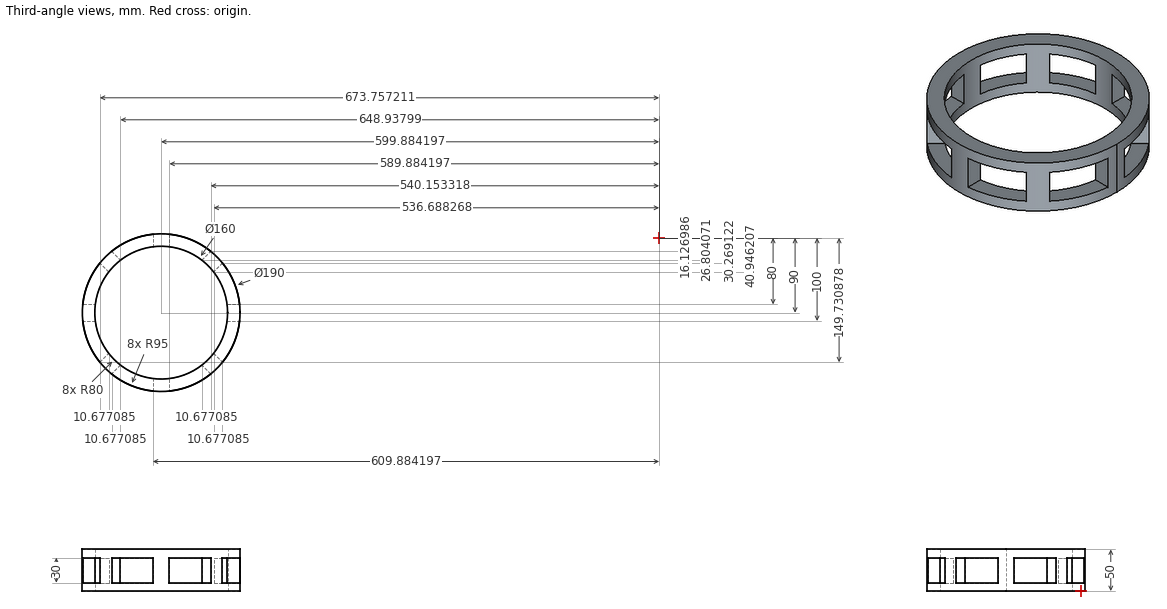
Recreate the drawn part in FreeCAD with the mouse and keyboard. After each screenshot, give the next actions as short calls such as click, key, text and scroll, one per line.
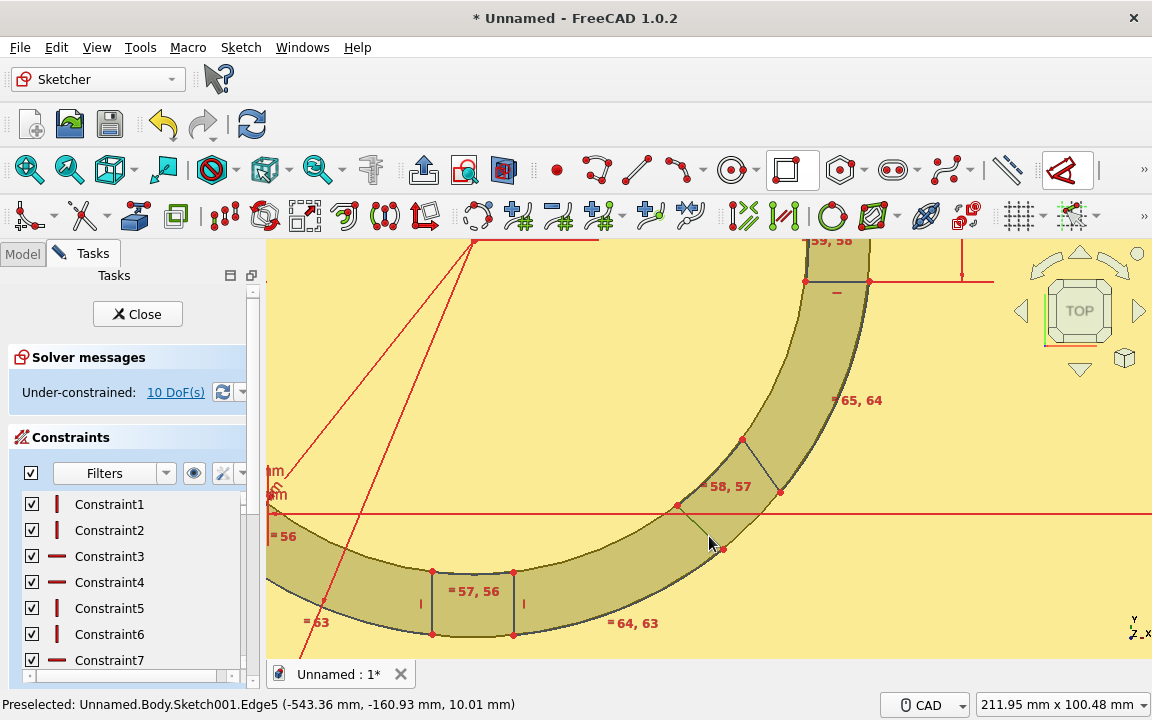
key(l)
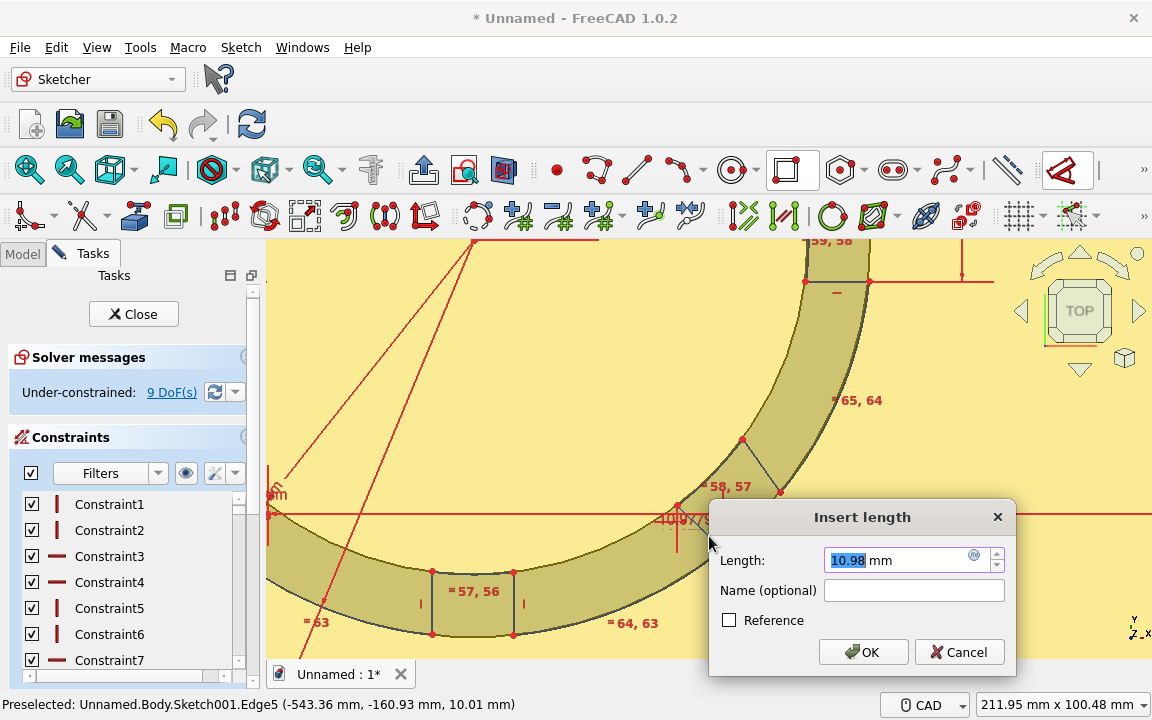
text(10.677085)
key(Return)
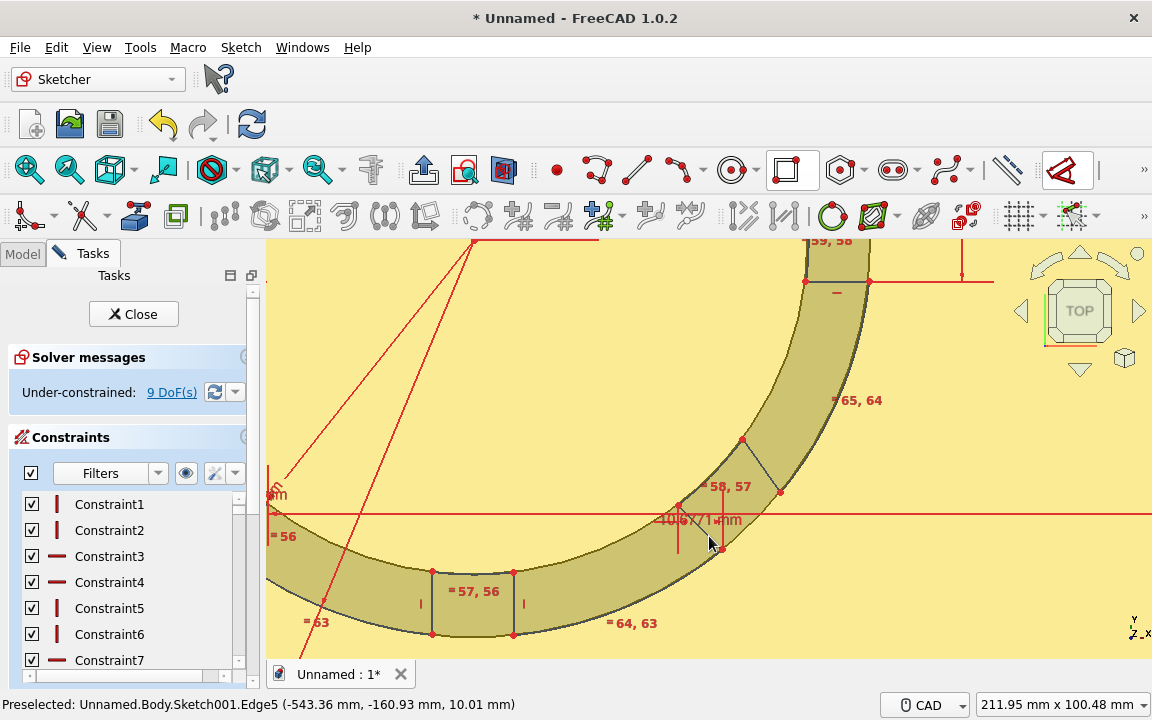
click(754, 455)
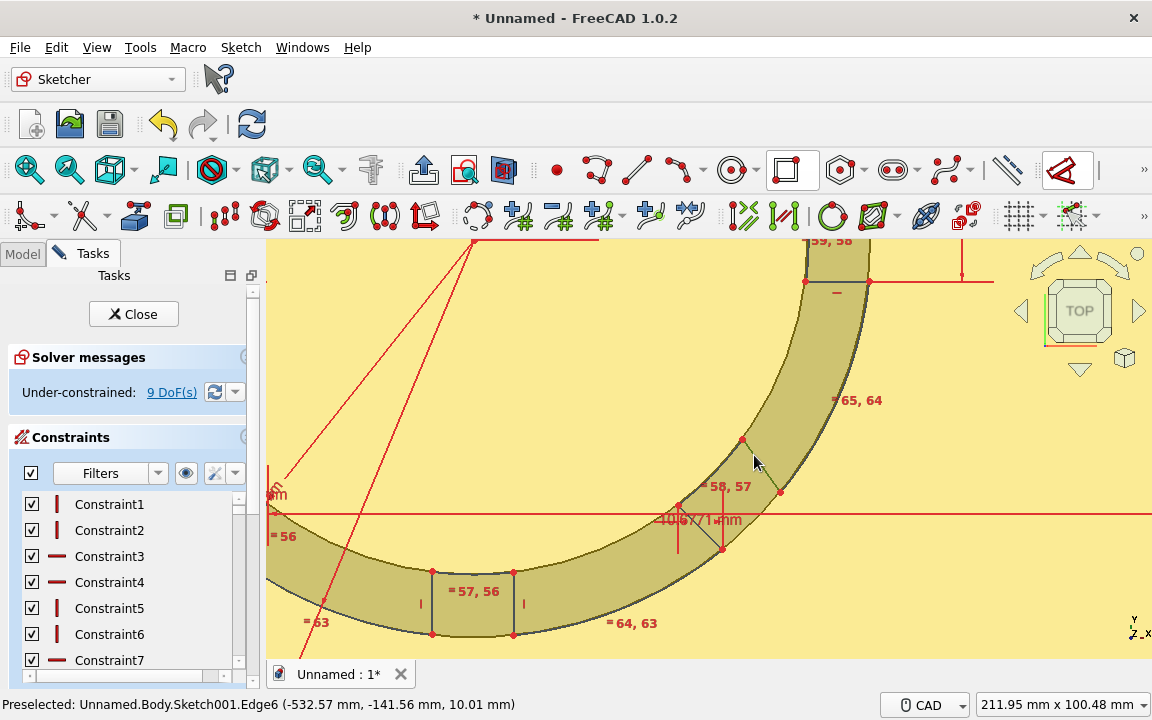
key(l)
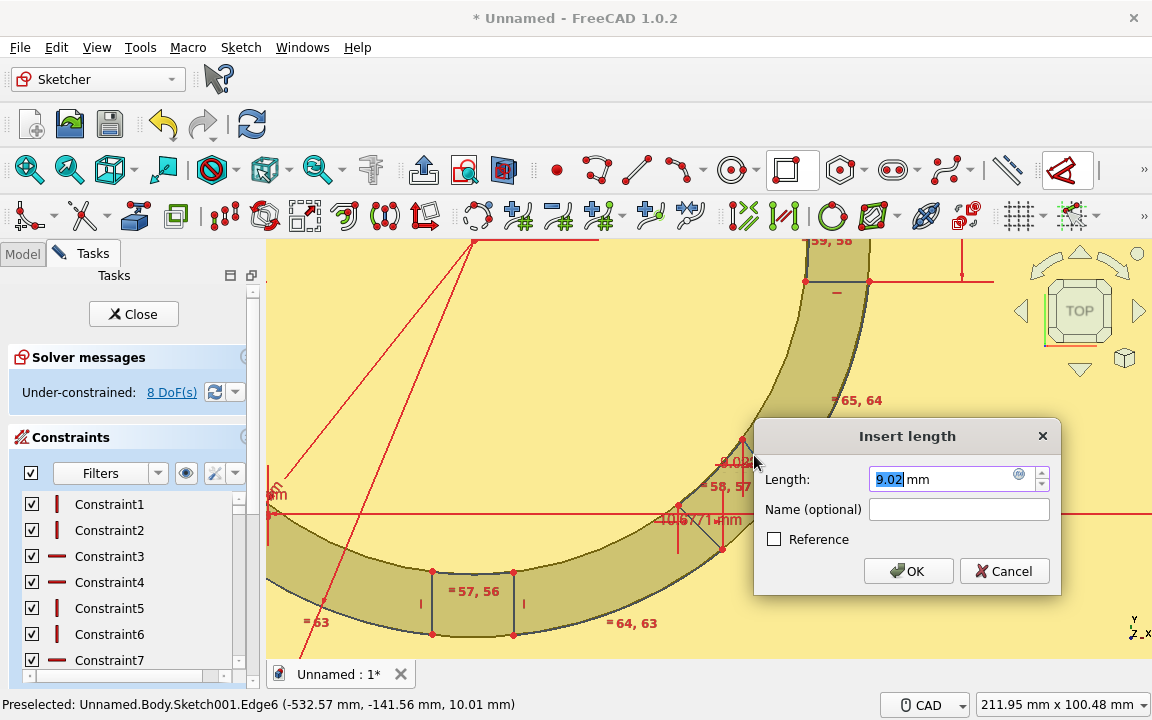
text(10.677085)
key(Return)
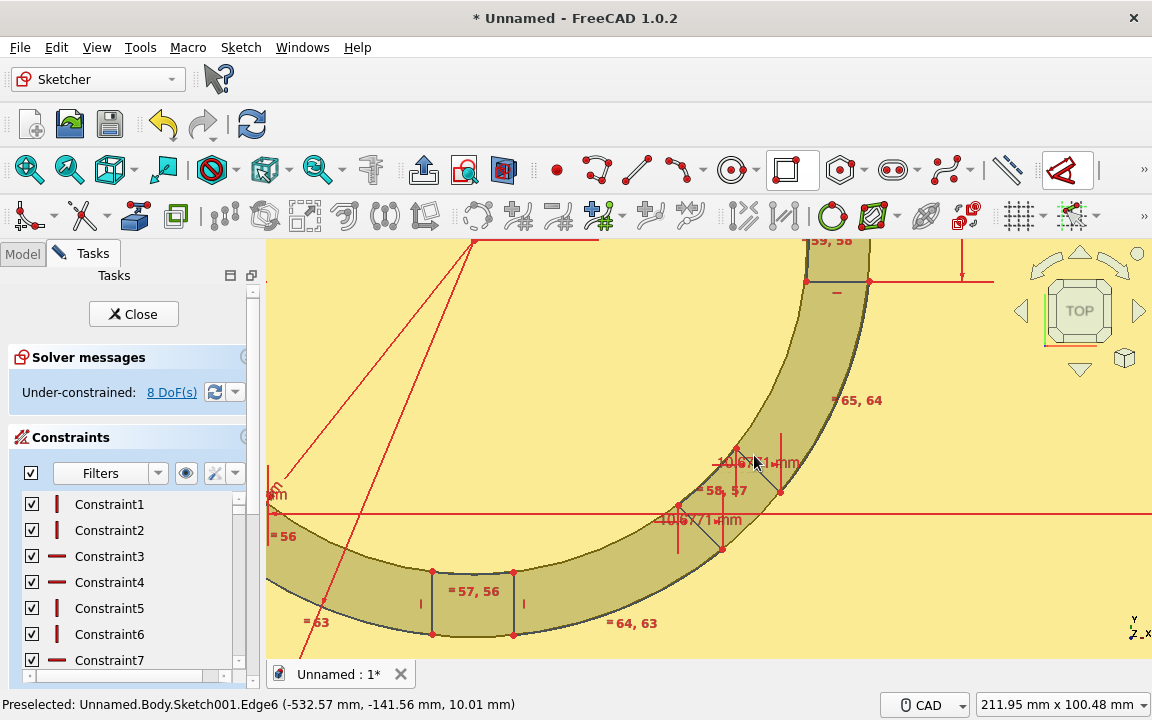
scroll(713, 539, down, 6)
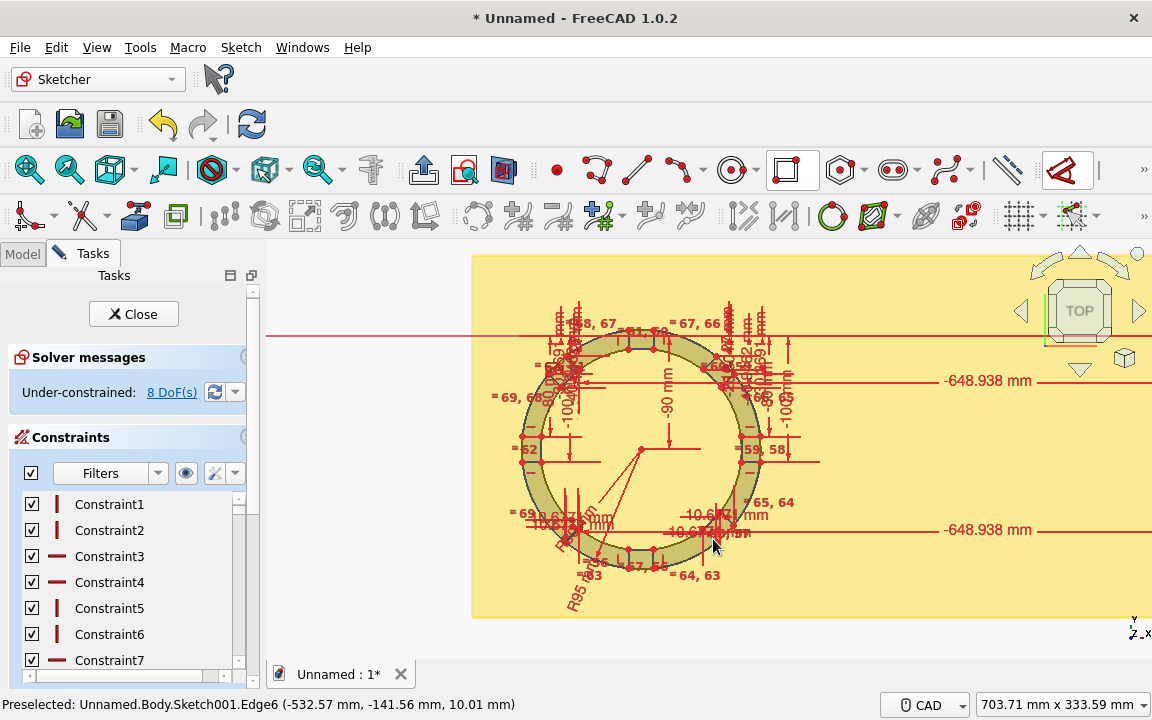
scroll(565, 541, up, 12)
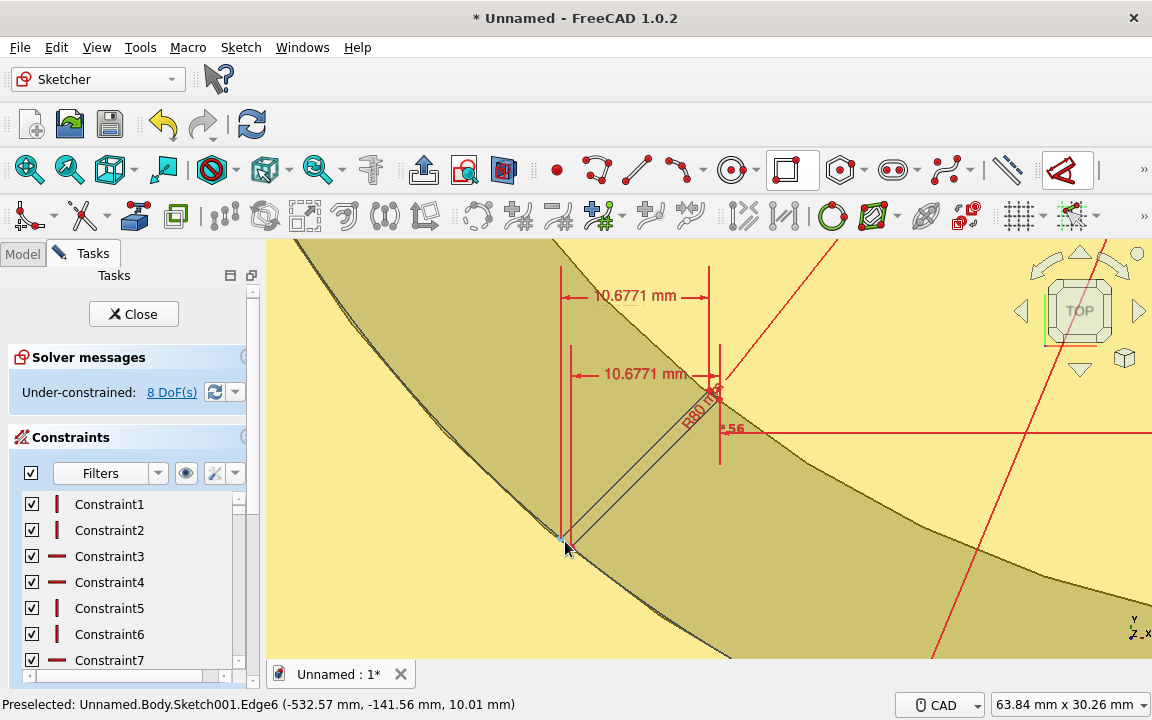
click(561, 538)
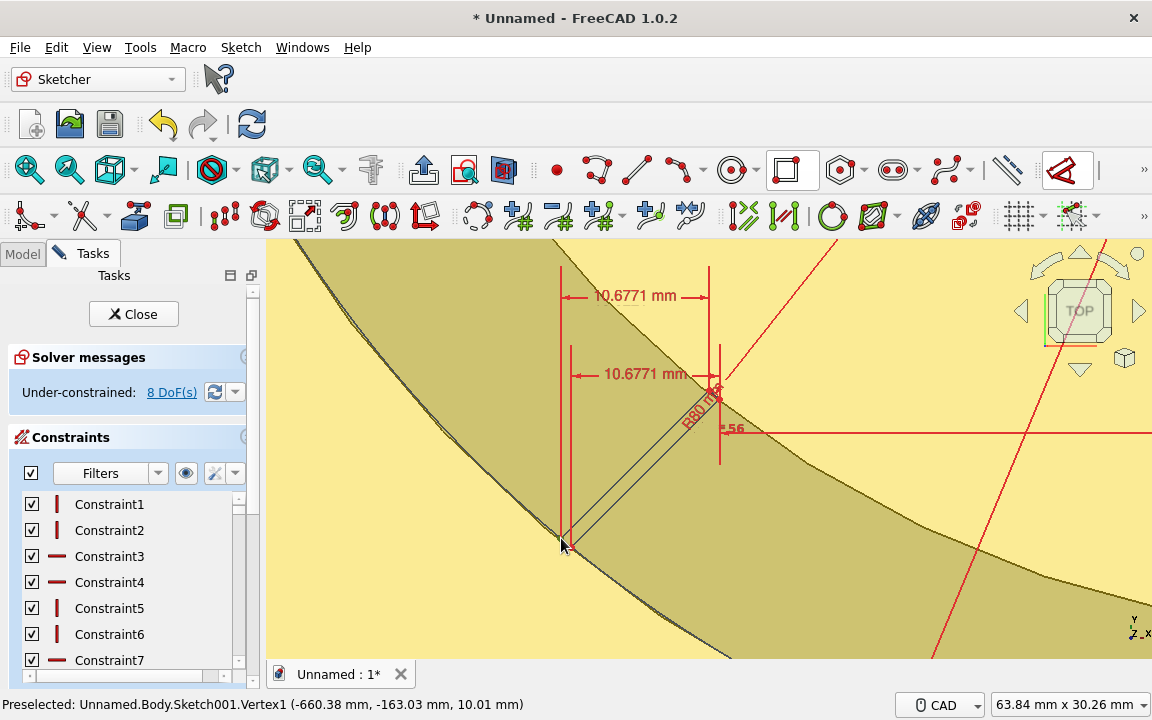
key(l)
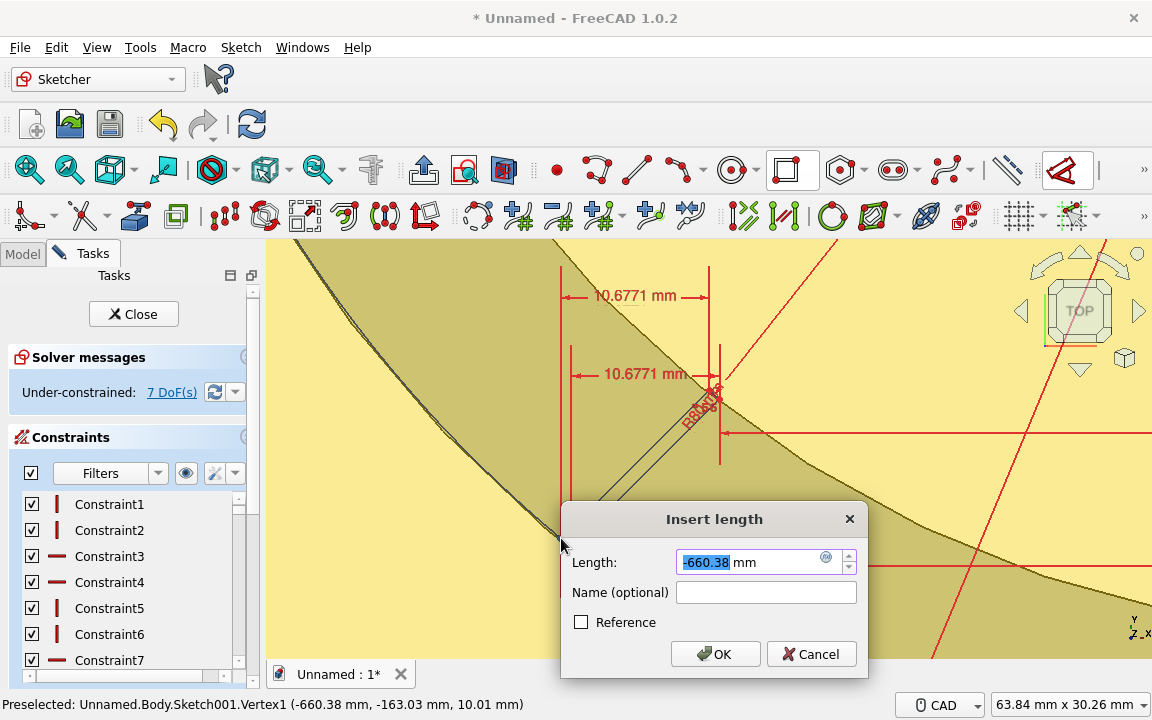
text(-673.757211)
key(Return)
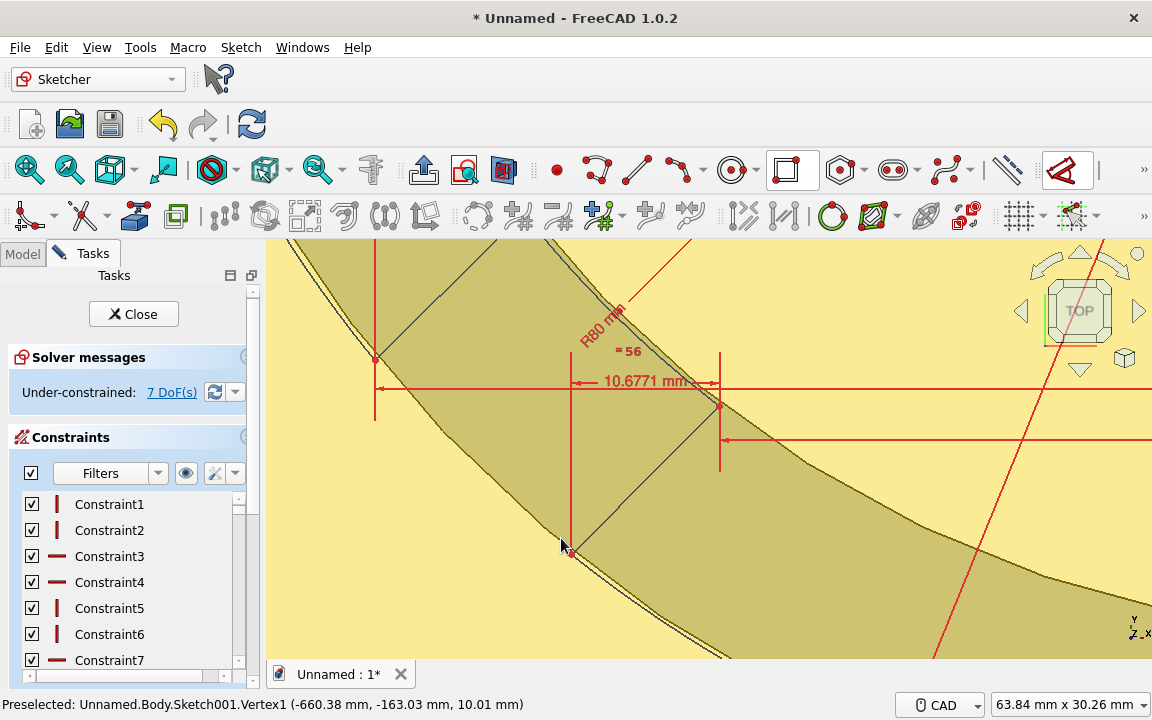
scroll(565, 541, down, 12)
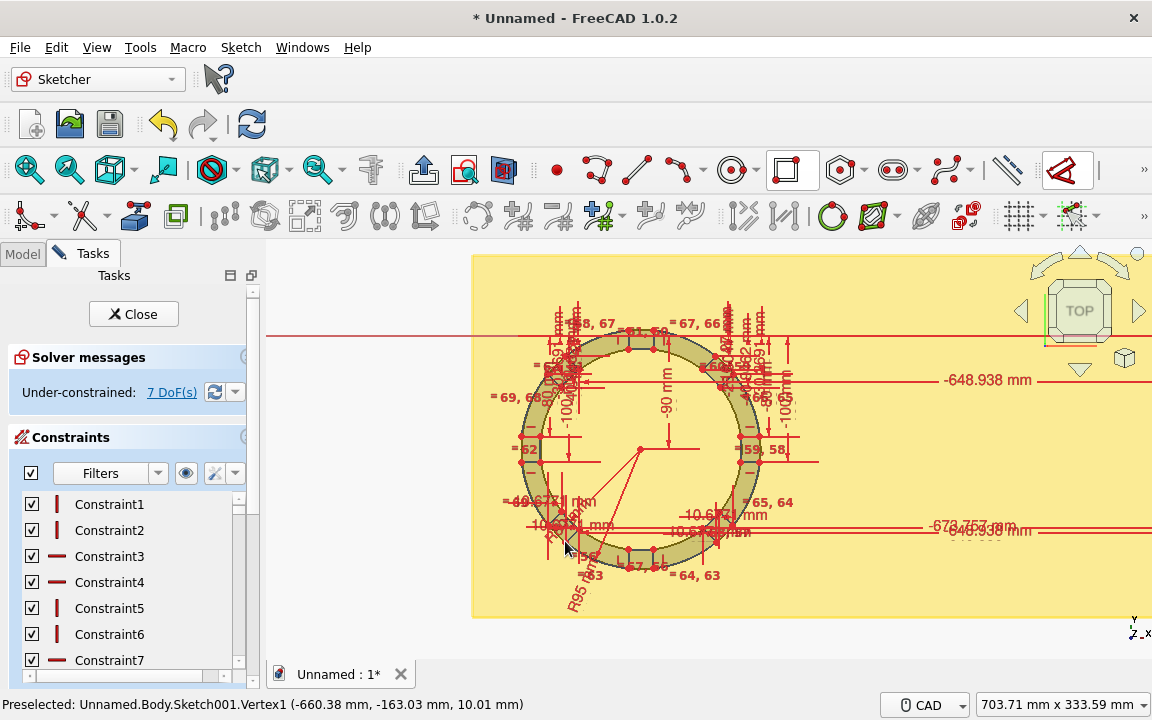
click(548, 525)